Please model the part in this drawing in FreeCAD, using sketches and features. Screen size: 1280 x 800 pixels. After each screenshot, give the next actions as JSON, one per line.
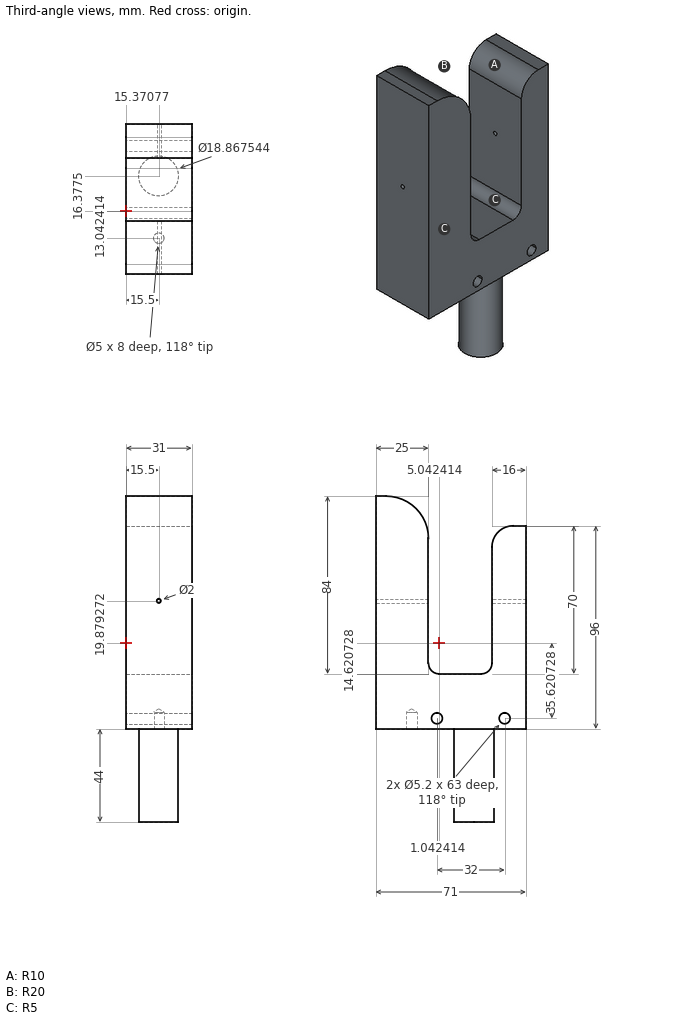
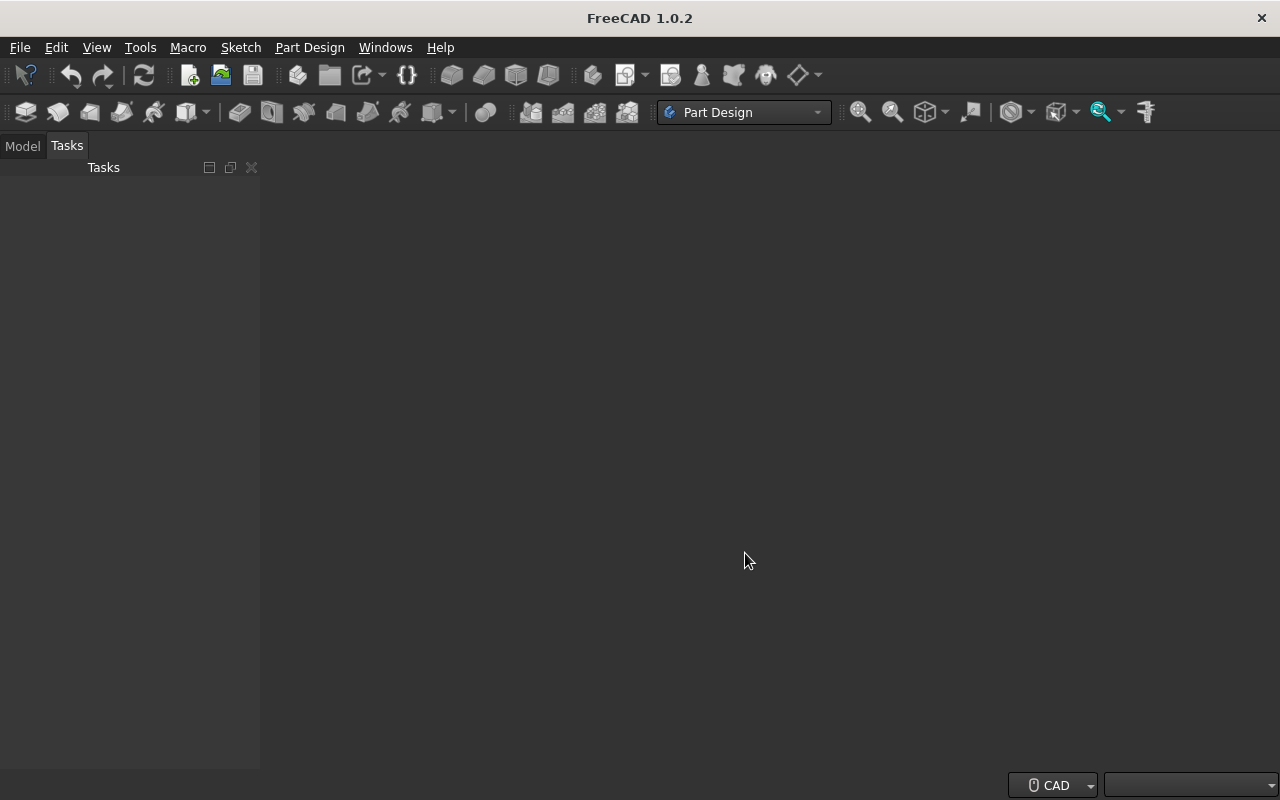
{"action": "left_click", "coordinate": [190, 76]}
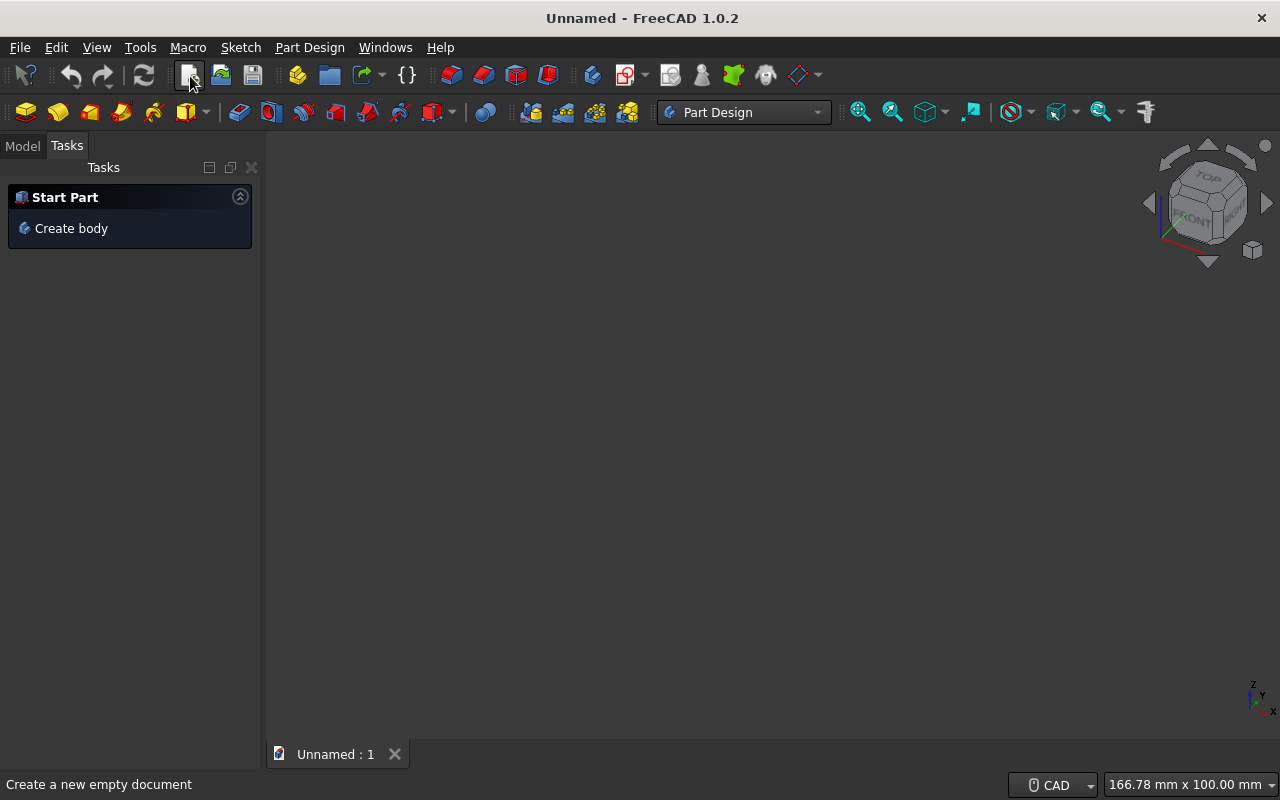
{"action": "left_click", "coordinate": [626, 76]}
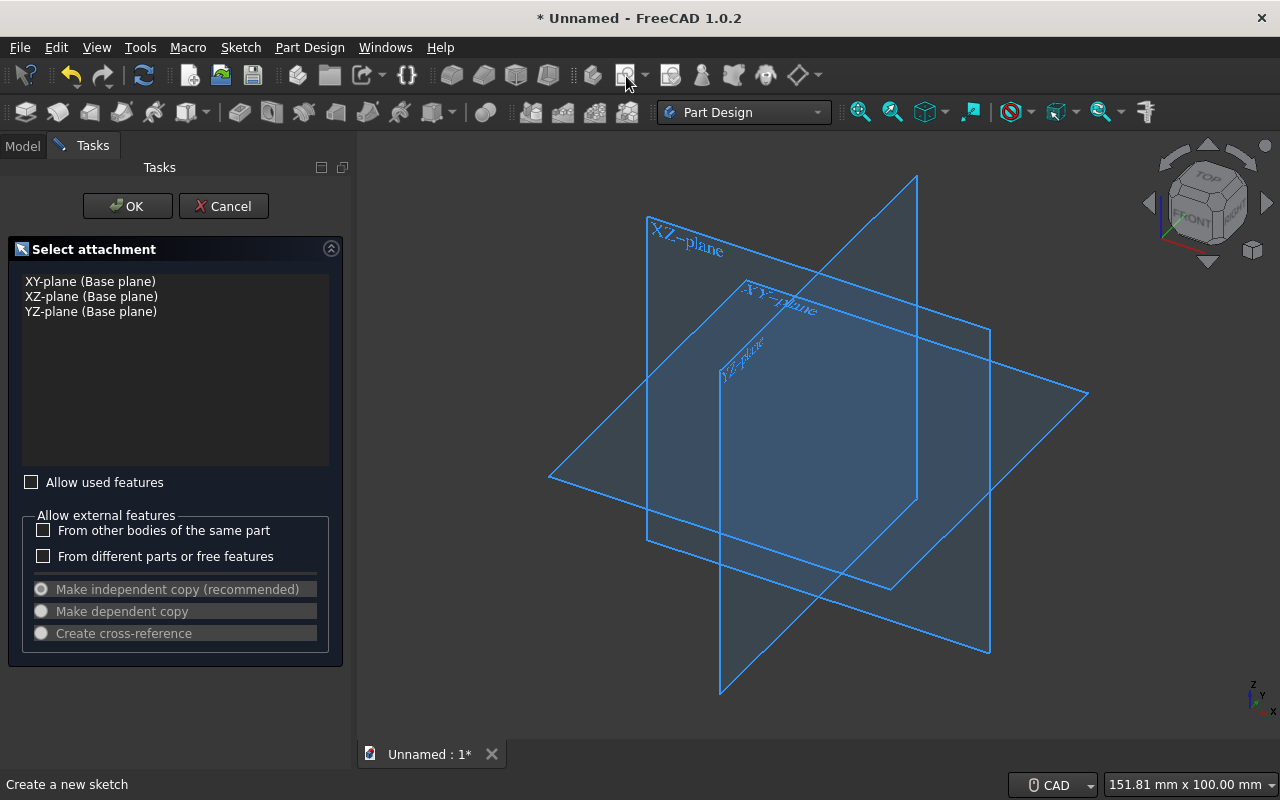
{"action": "left_click", "coordinate": [82, 312]}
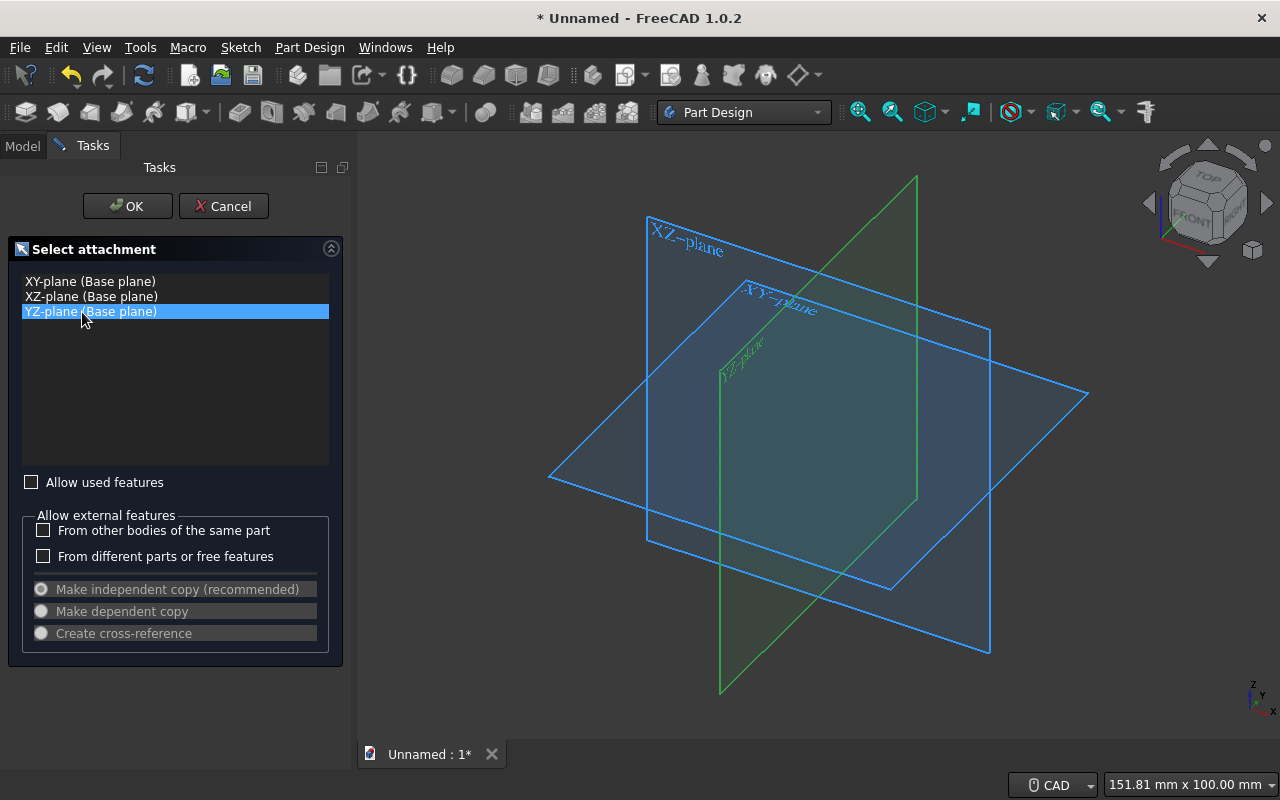
{"action": "left_click", "coordinate": [128, 206]}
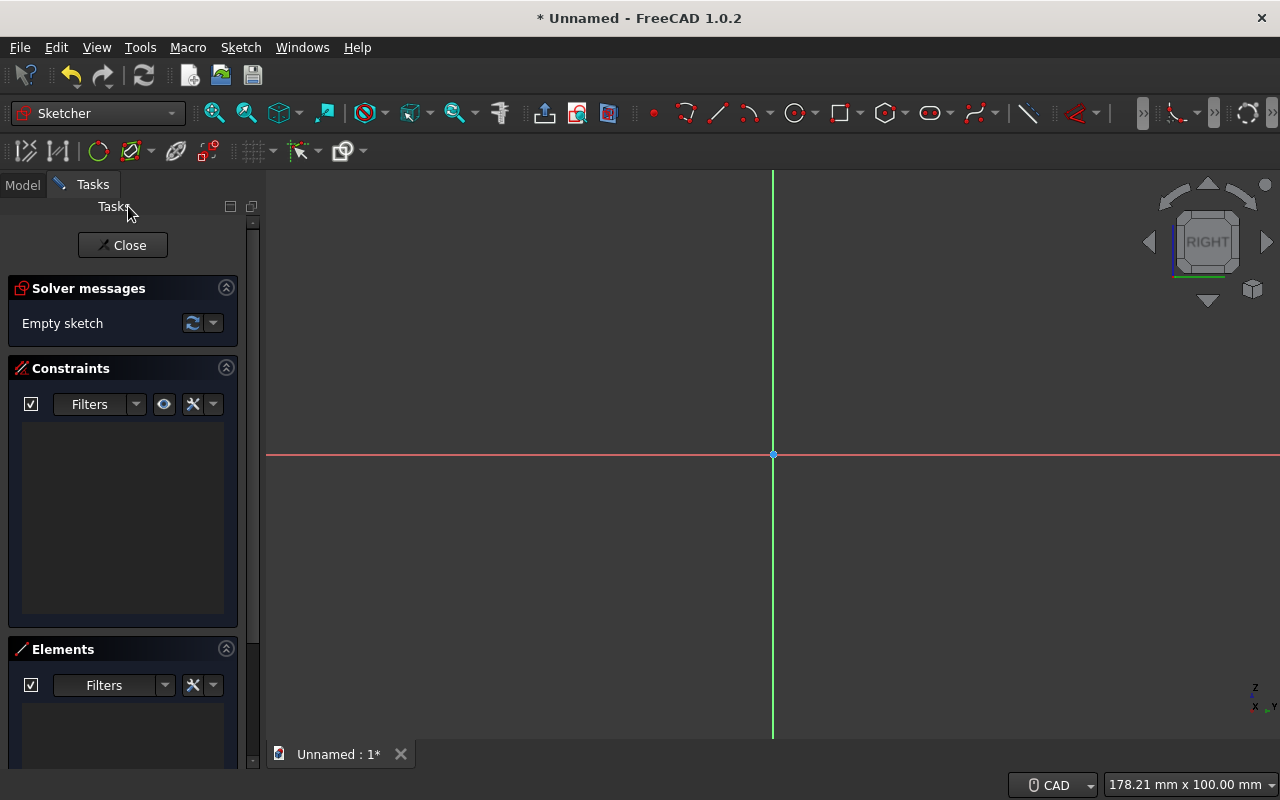
{"action": "scroll", "coordinate": [583, 554], "scroll_direction": "down", "scroll_amount": 3}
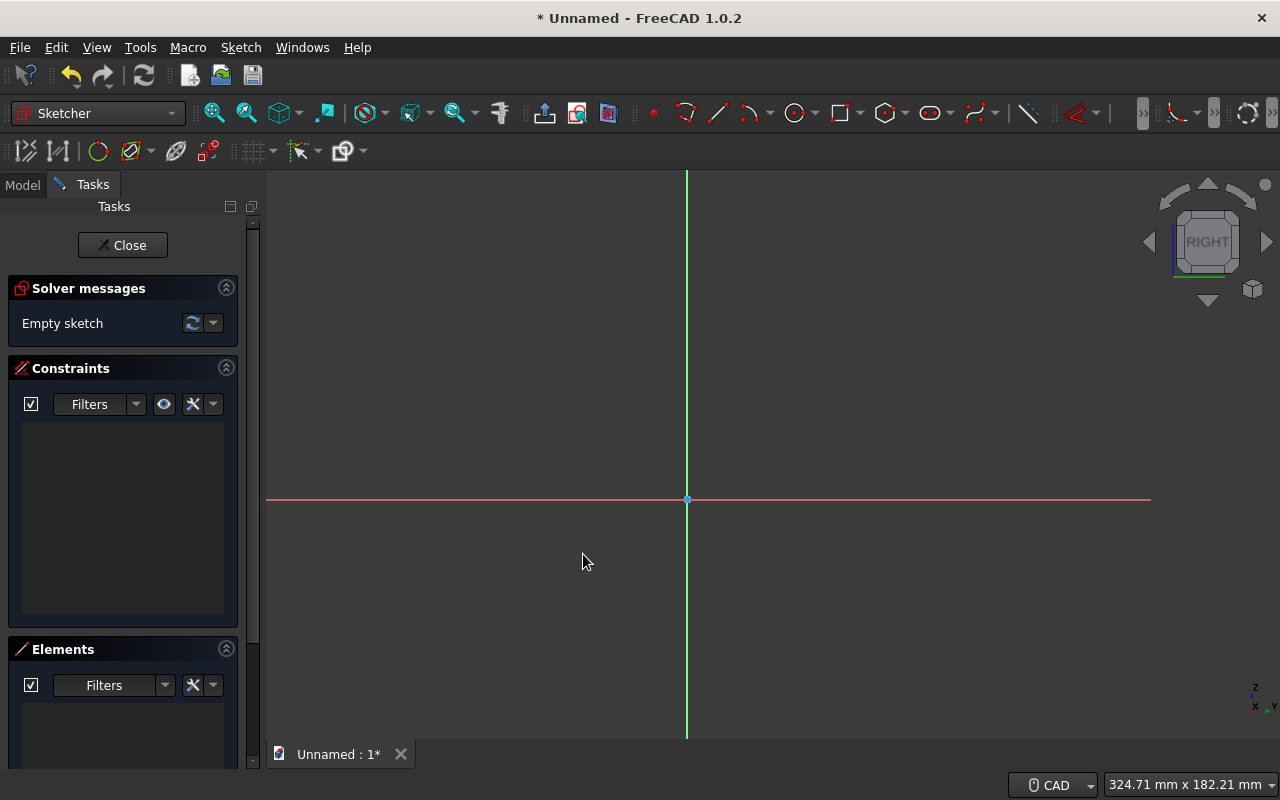
{"action": "left_click", "coordinate": [686, 114]}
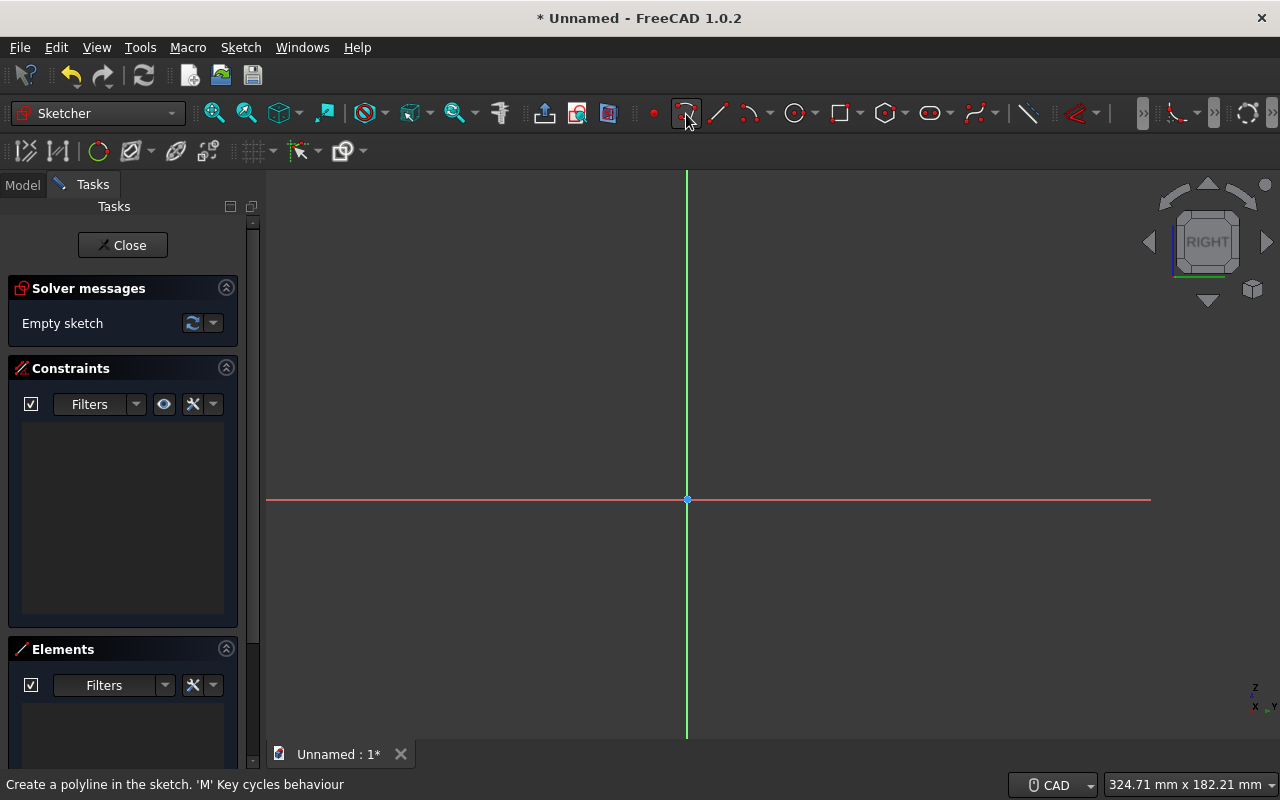
{"action": "left_click", "coordinate": [672, 545]}
{"action": "left_click", "coordinate": [672, 283]}
{"action": "left_click", "coordinate": [594, 283]}
{"action": "left_click", "coordinate": [594, 627]}
{"action": "left_click", "coordinate": [815, 627]}
{"action": "left_click", "coordinate": [815, 327]}
{"action": "left_click", "coordinate": [765, 327]}
{"action": "left_click", "coordinate": [765, 545]}
{"action": "left_click", "coordinate": [672, 546]}
{"action": "key", "text": "Escape"}
{"action": "key", "text": "Escape"}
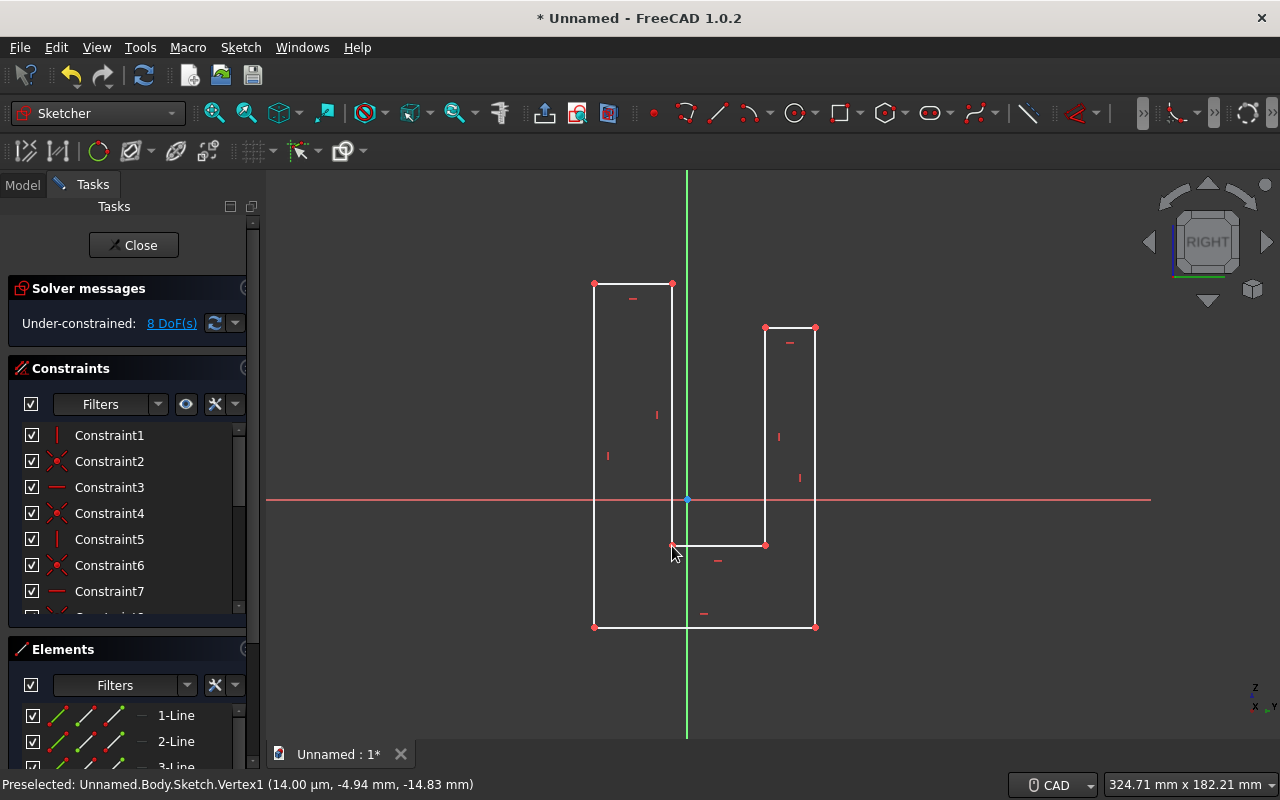
{"action": "left_click", "coordinate": [672, 467]}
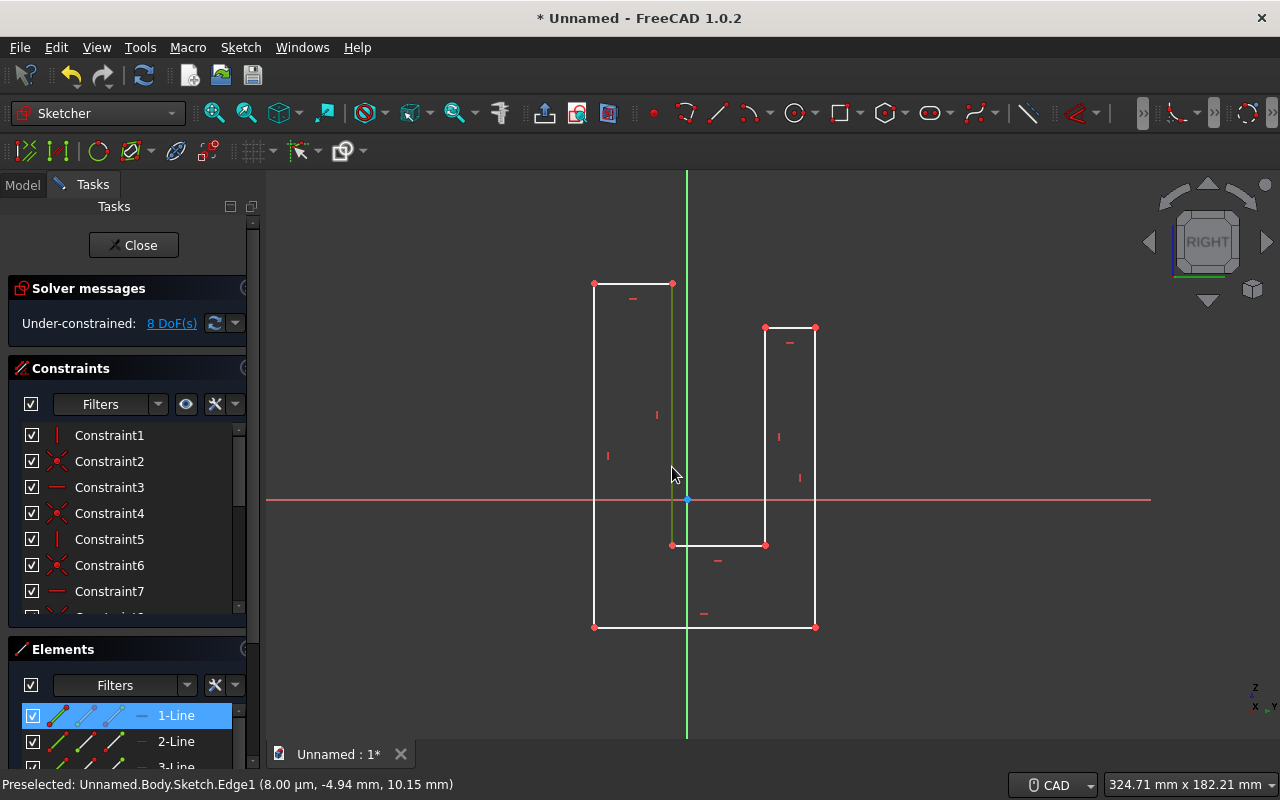
{"action": "key", "text": "i"}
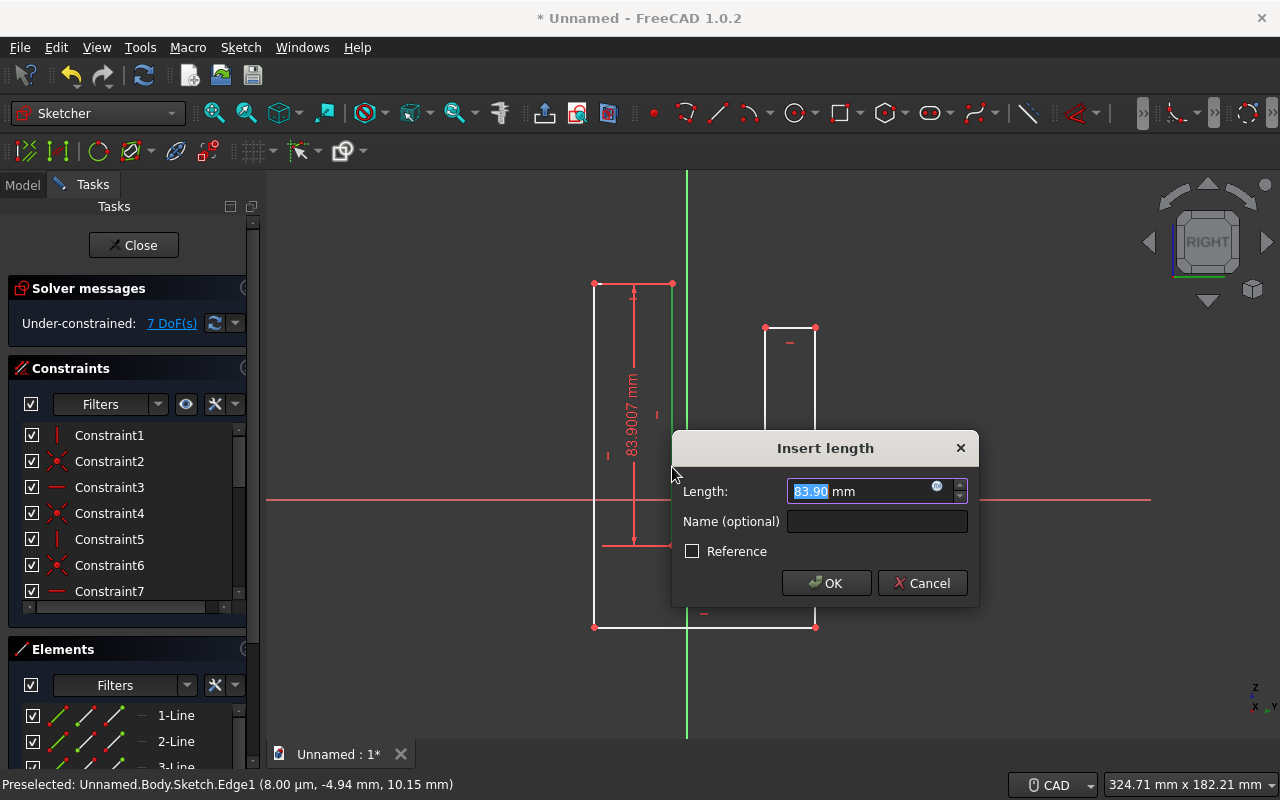
{"action": "type", "text": "84"}
{"action": "key", "text": "Return"}